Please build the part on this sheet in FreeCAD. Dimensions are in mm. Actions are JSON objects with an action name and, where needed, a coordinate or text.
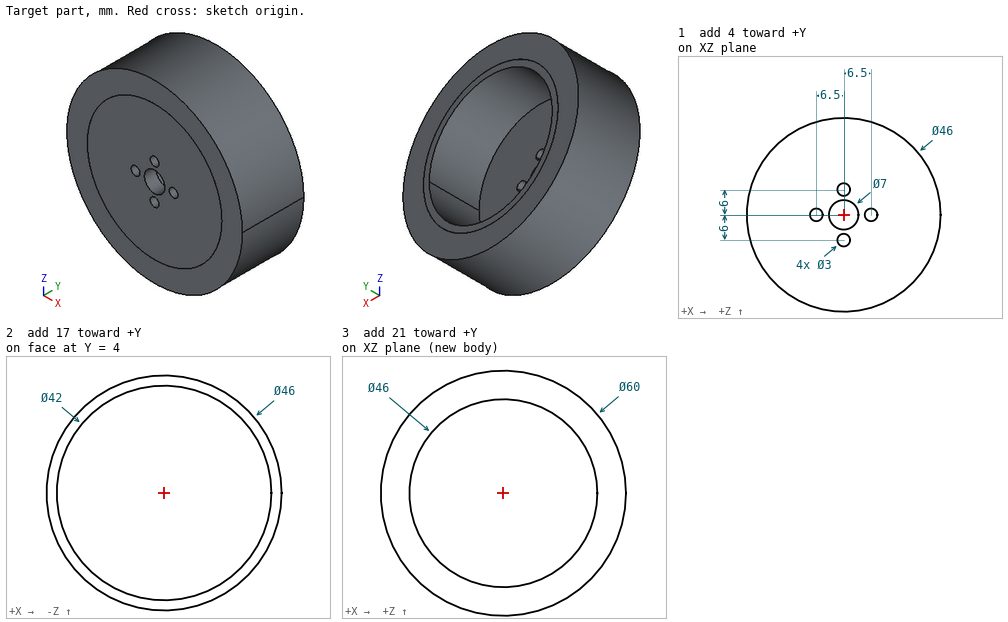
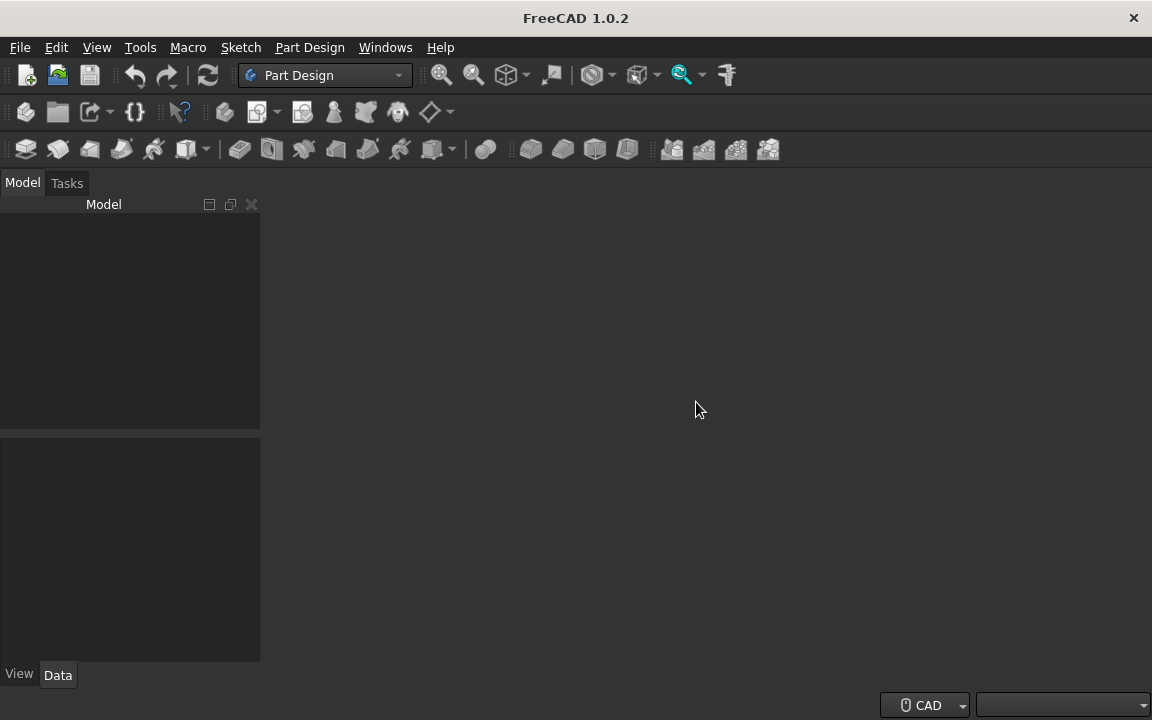
{"action": "left_click", "coordinate": [26, 76]}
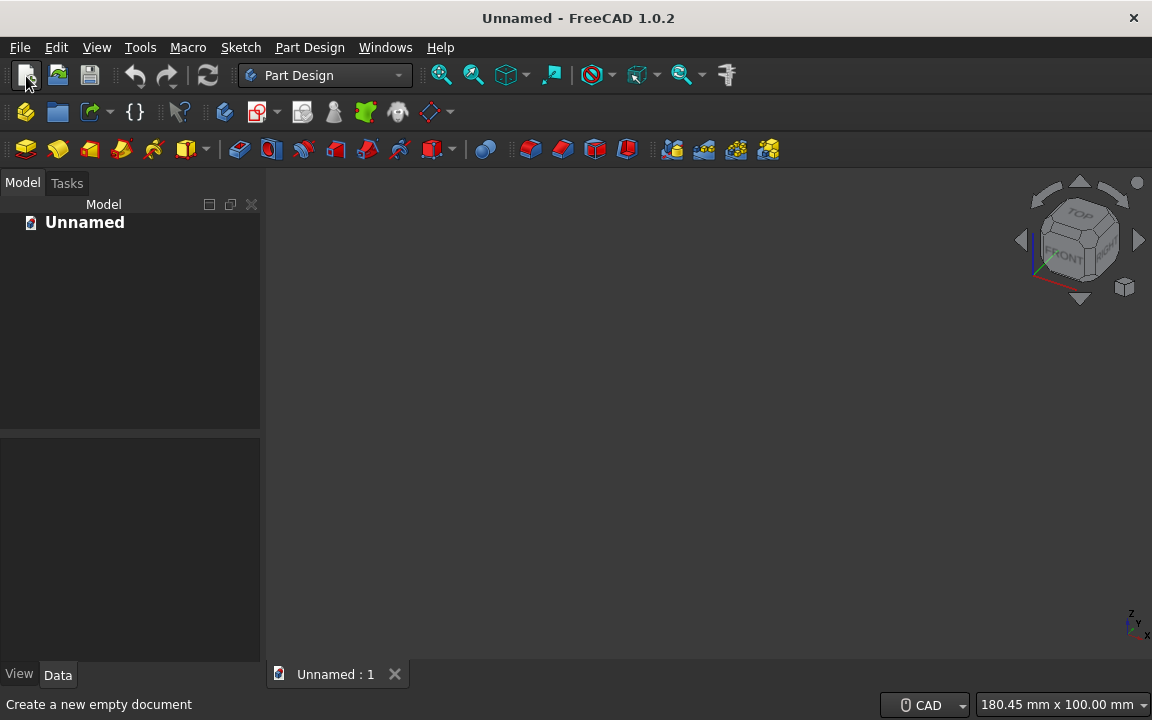
{"action": "left_click", "coordinate": [258, 112]}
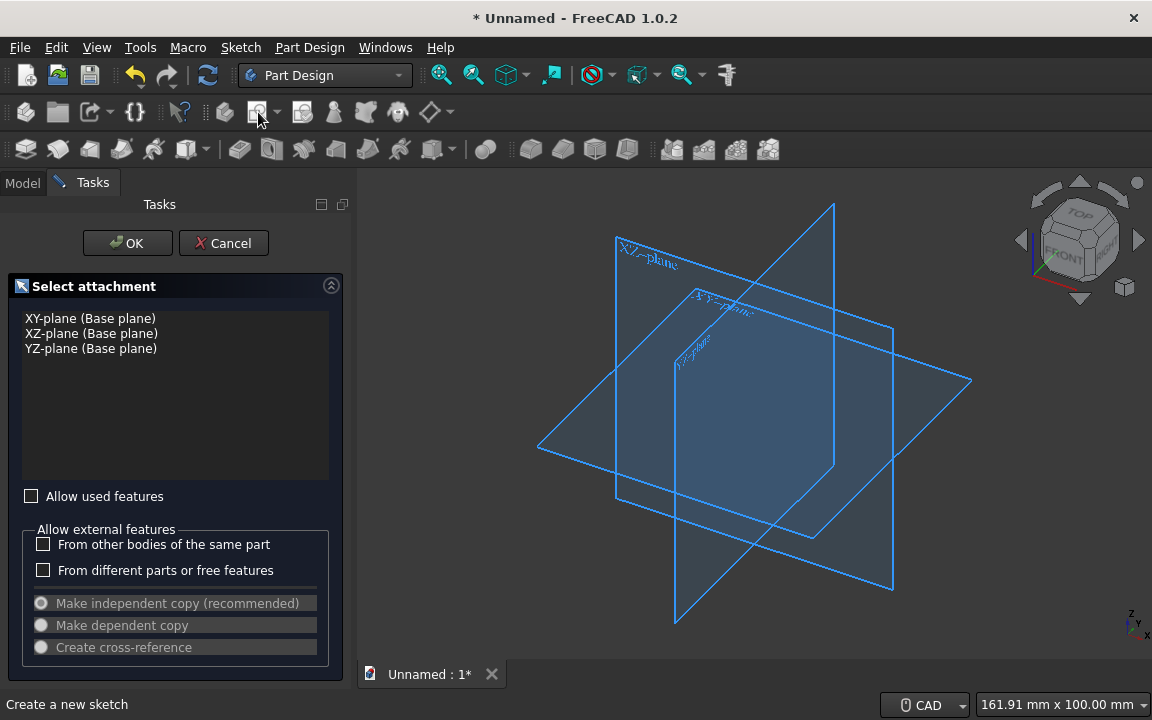
{"action": "left_click", "coordinate": [82, 334]}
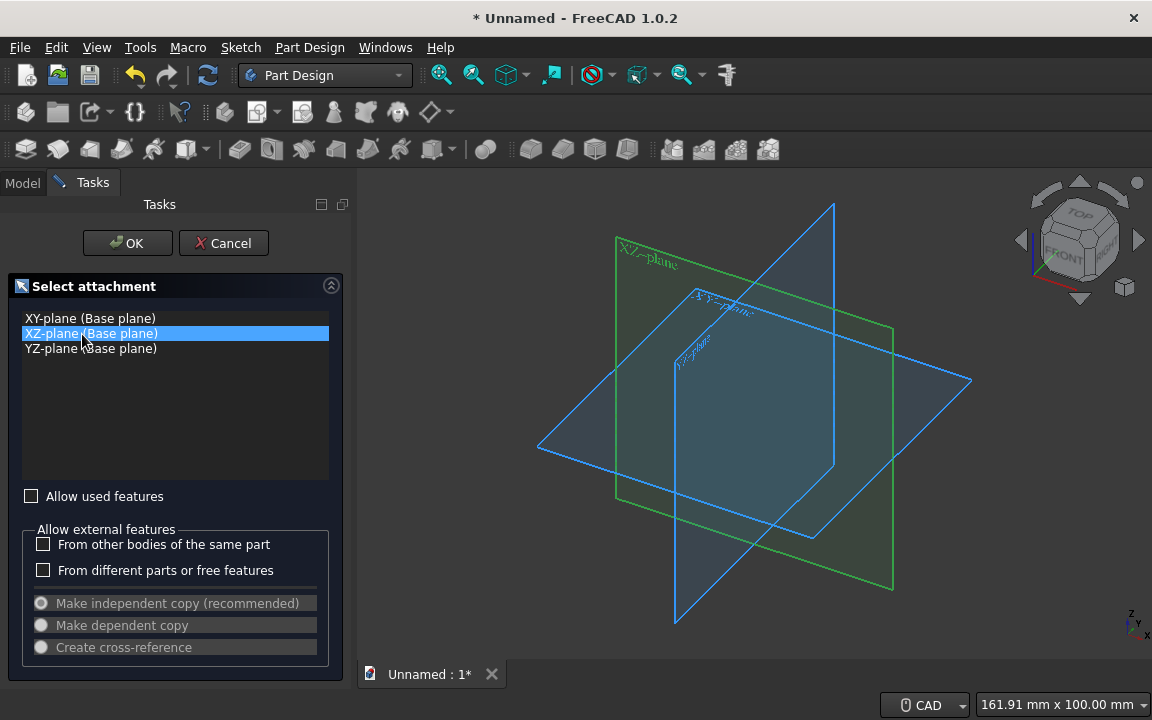
{"action": "left_click", "coordinate": [128, 243]}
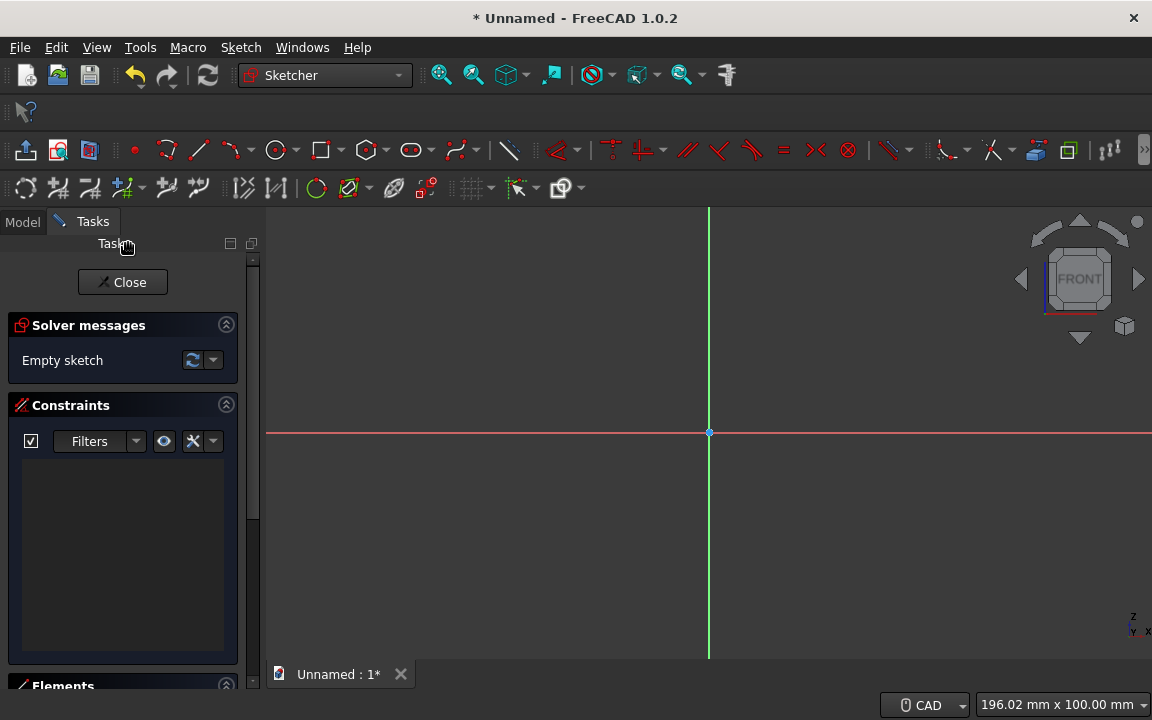
{"action": "left_click", "coordinate": [276, 150]}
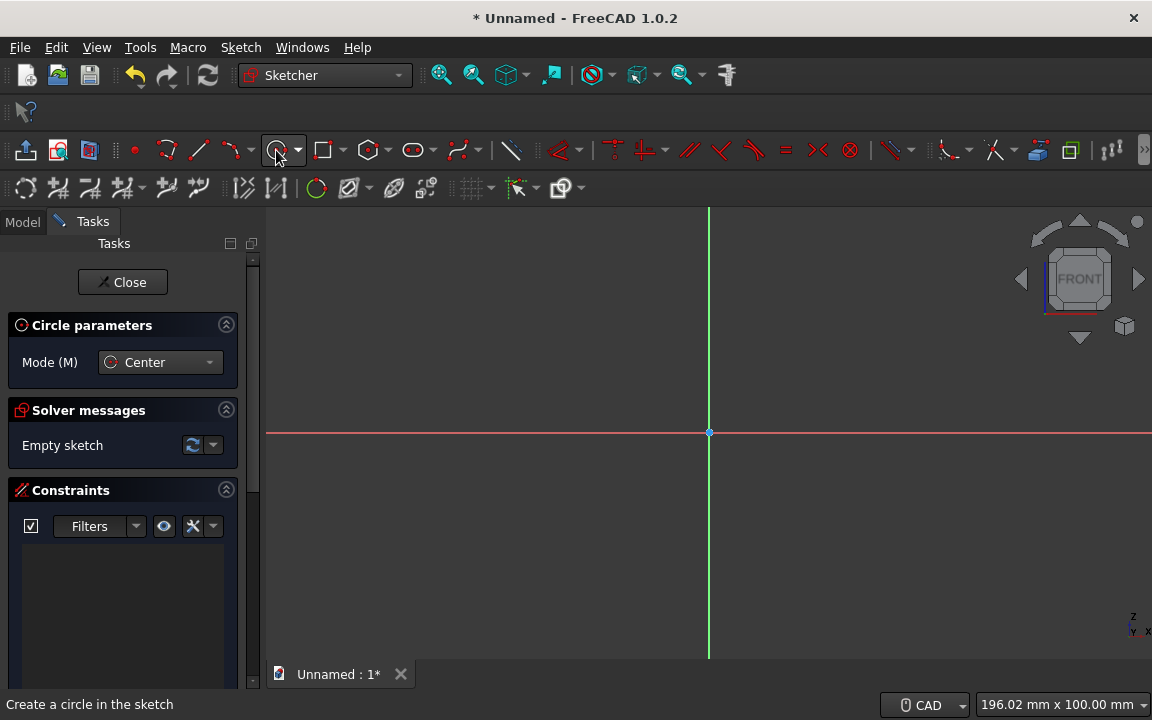
{"action": "left_click", "coordinate": [709, 433]}
{"action": "left_click", "coordinate": [783, 359]}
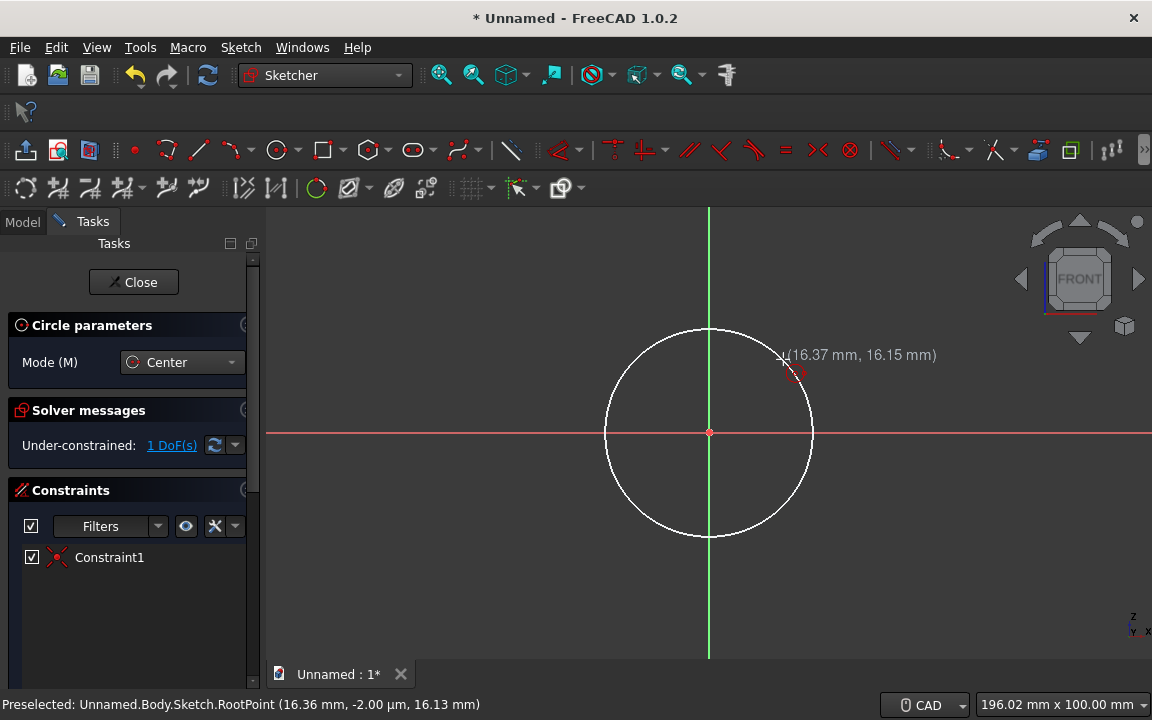
{"action": "scroll", "coordinate": [709, 460], "scroll_direction": "up", "scroll_amount": 7}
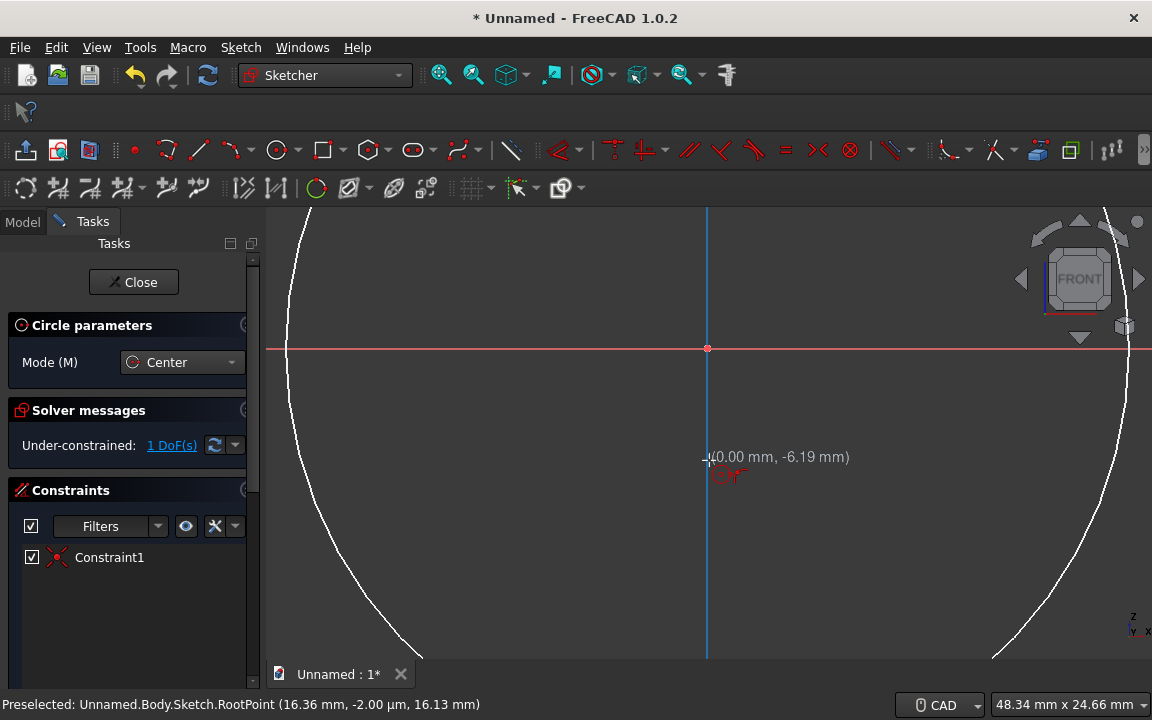
{"action": "scroll", "coordinate": [612, 469], "scroll_direction": "down", "scroll_amount": 6}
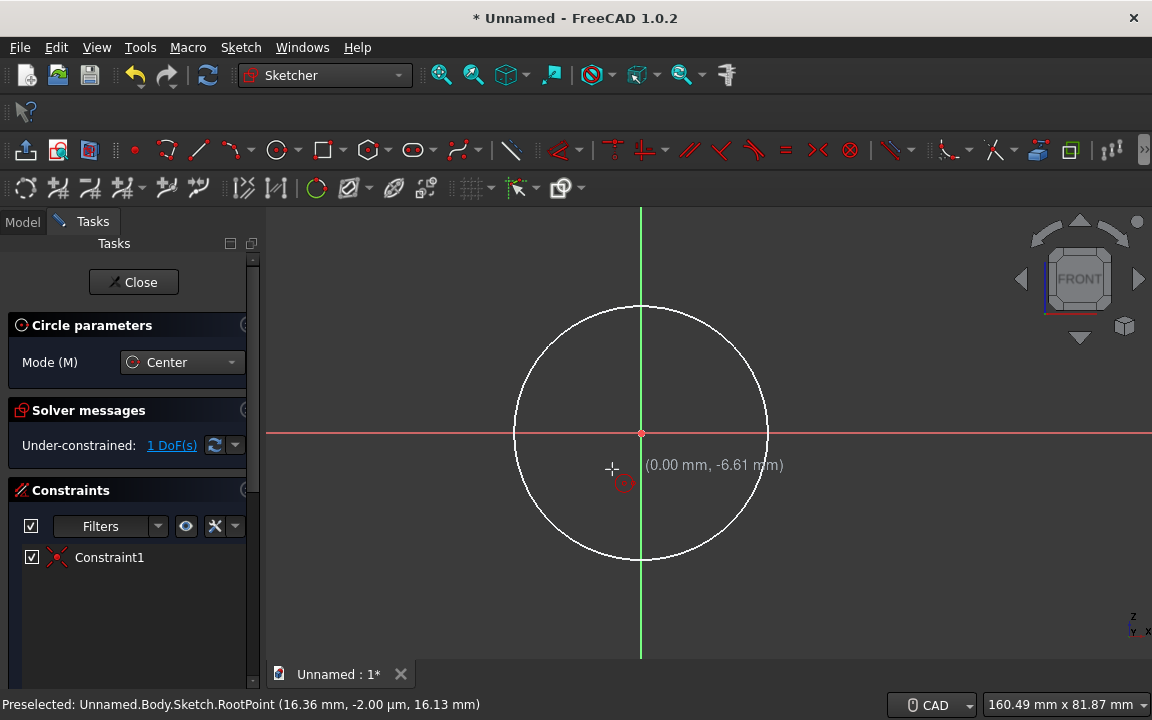
{"action": "left_click", "coordinate": [641, 466]}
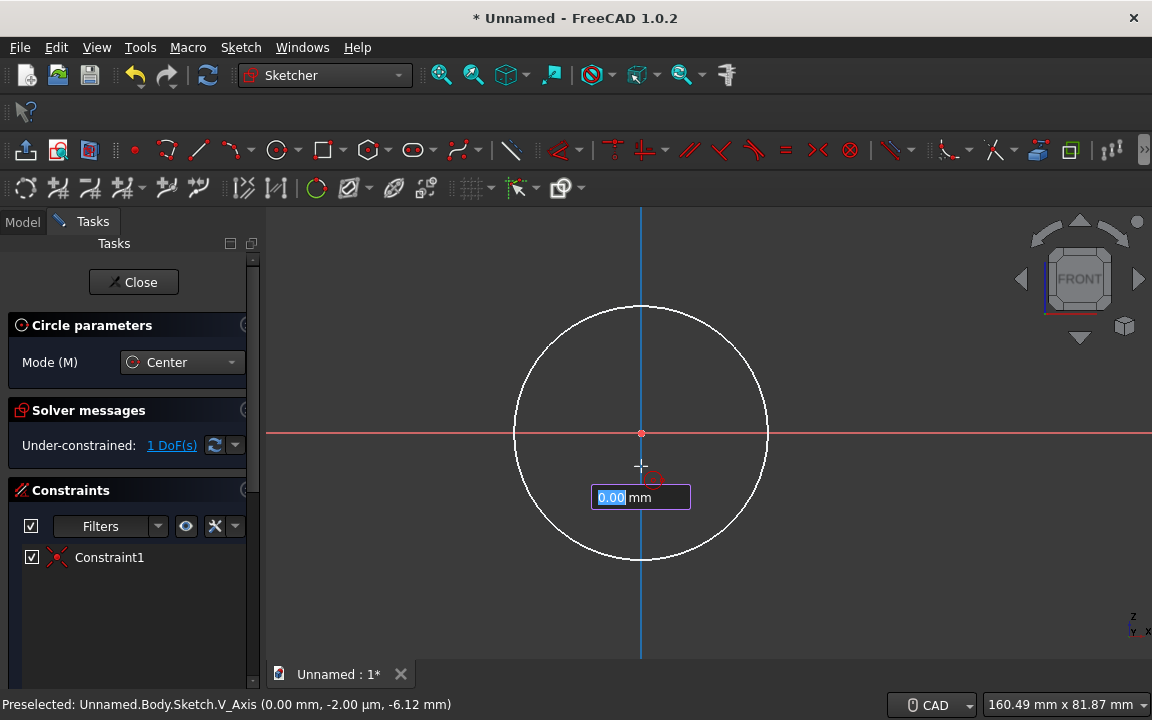
{"action": "scroll", "coordinate": [649, 463], "scroll_direction": "up", "scroll_amount": 4}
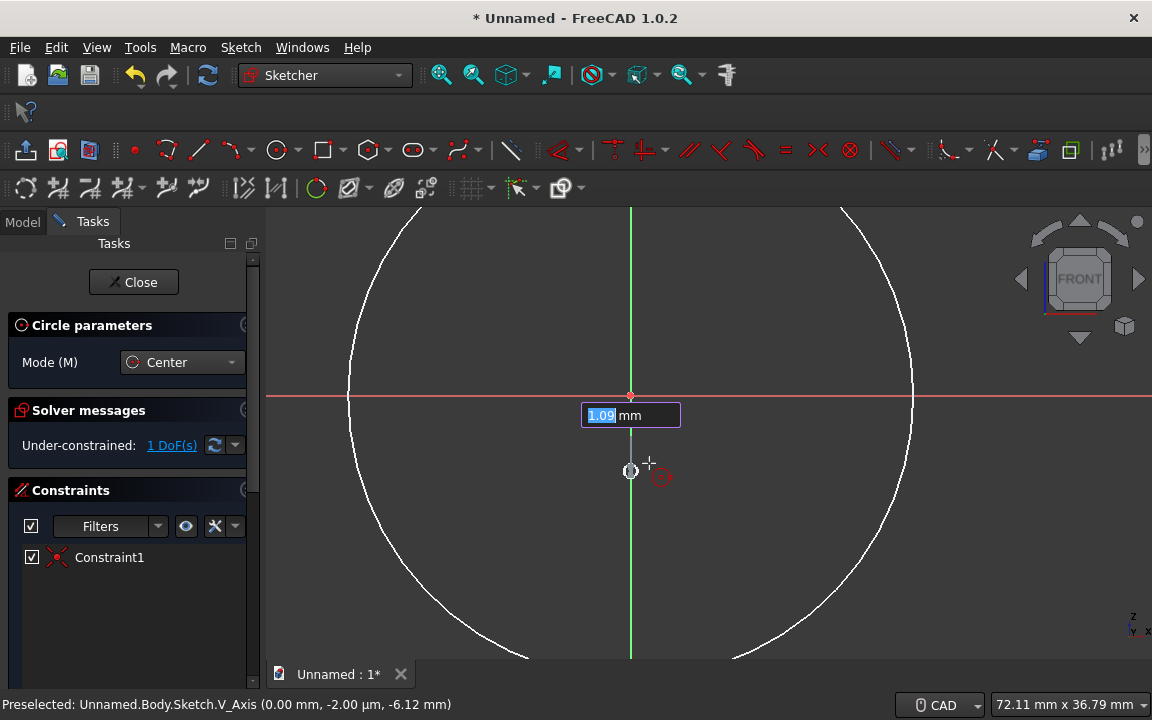
{"action": "left_click", "coordinate": [648, 463]}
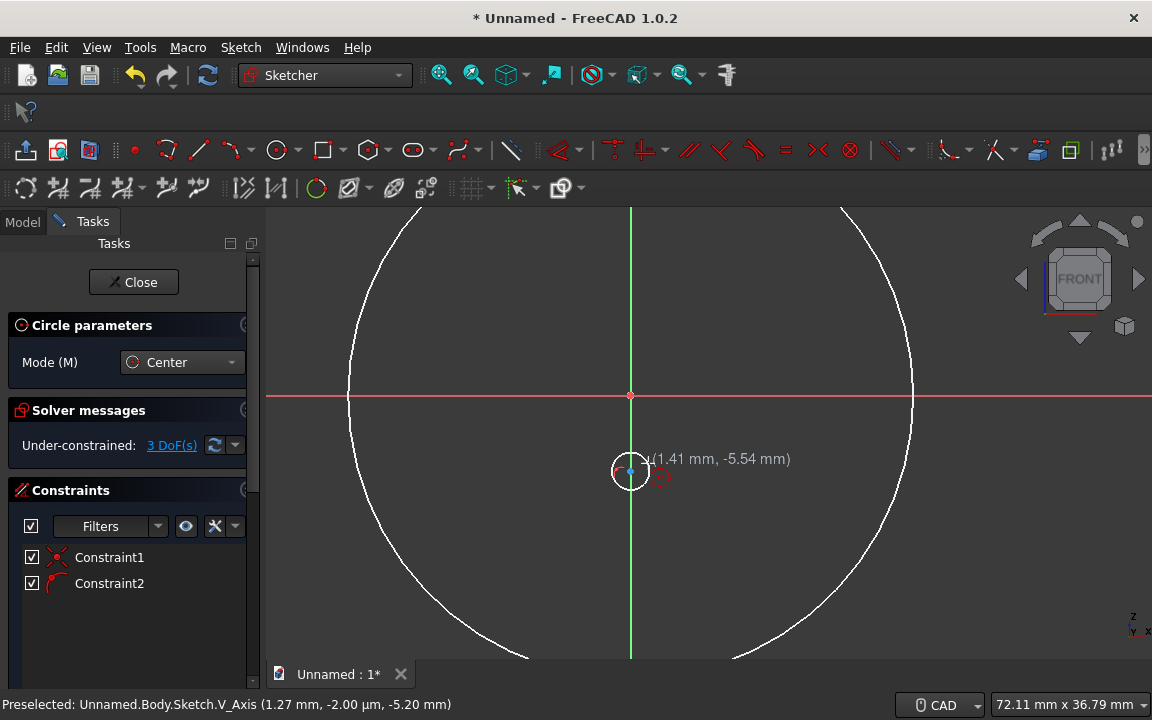
{"action": "scroll", "coordinate": [551, 396], "scroll_direction": "up", "scroll_amount": 2}